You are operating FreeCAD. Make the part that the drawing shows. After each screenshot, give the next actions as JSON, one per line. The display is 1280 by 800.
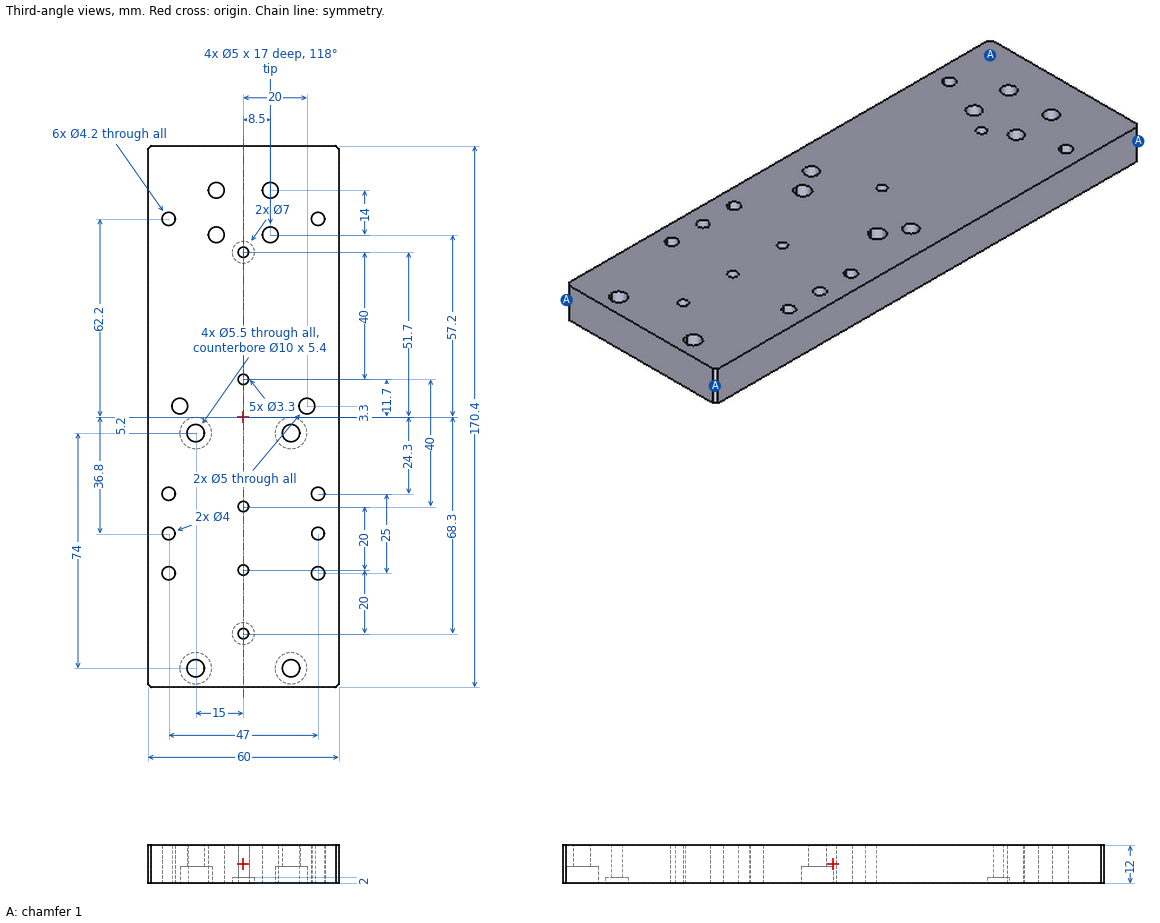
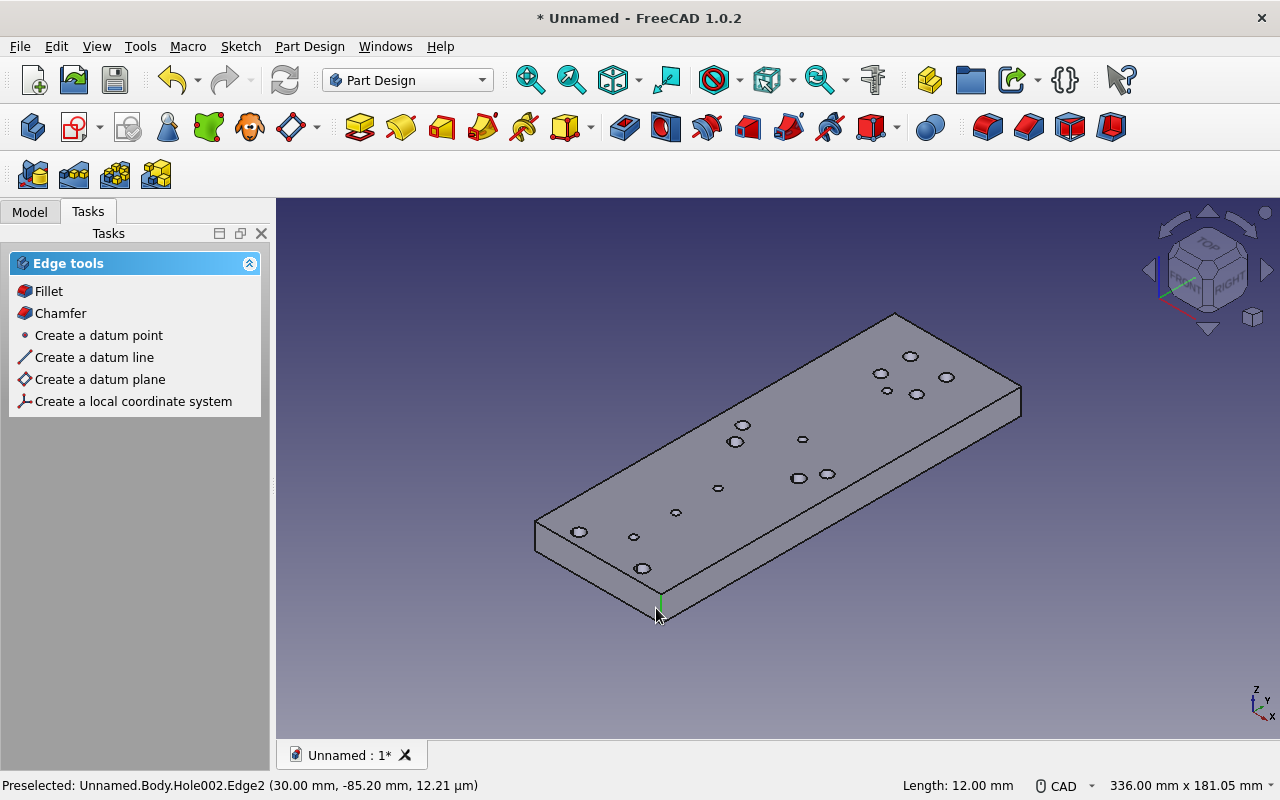
{"action": "key", "text": "1"}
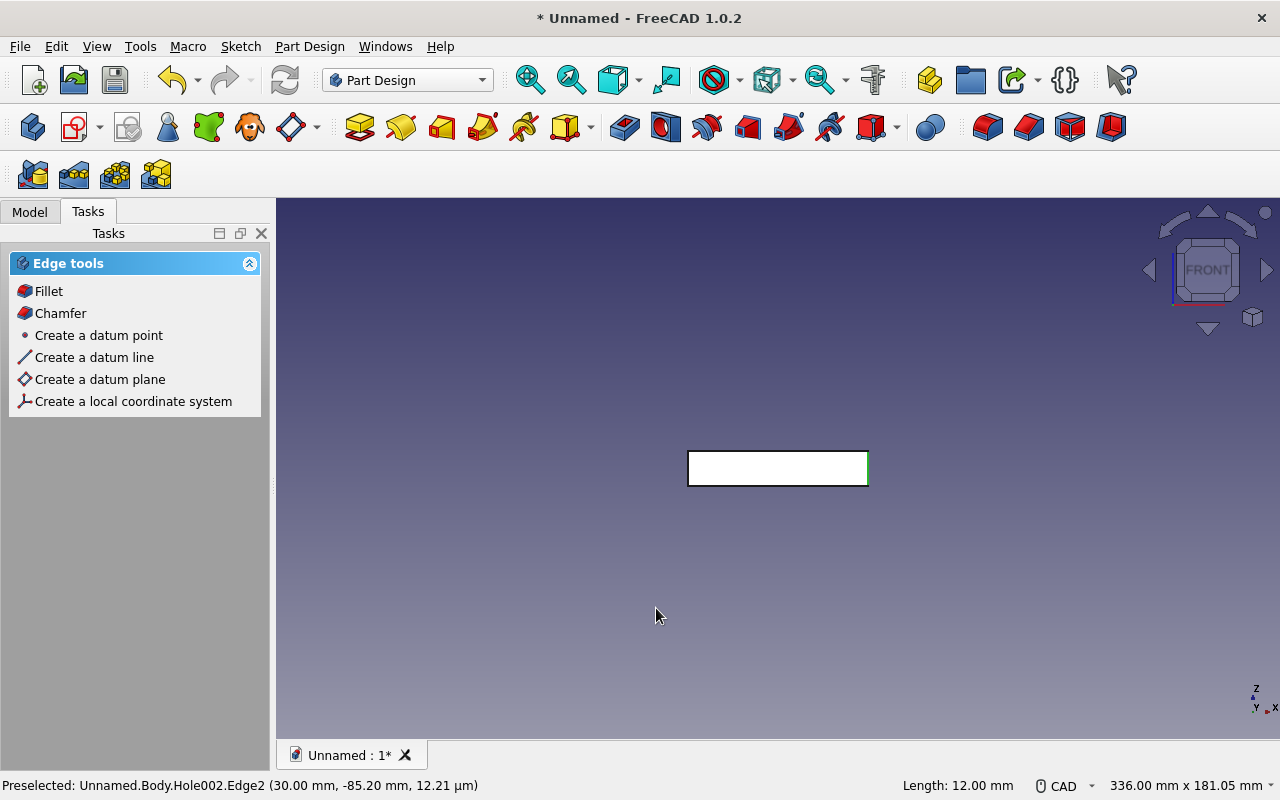
{"action": "left_click", "coordinate": [531, 80]}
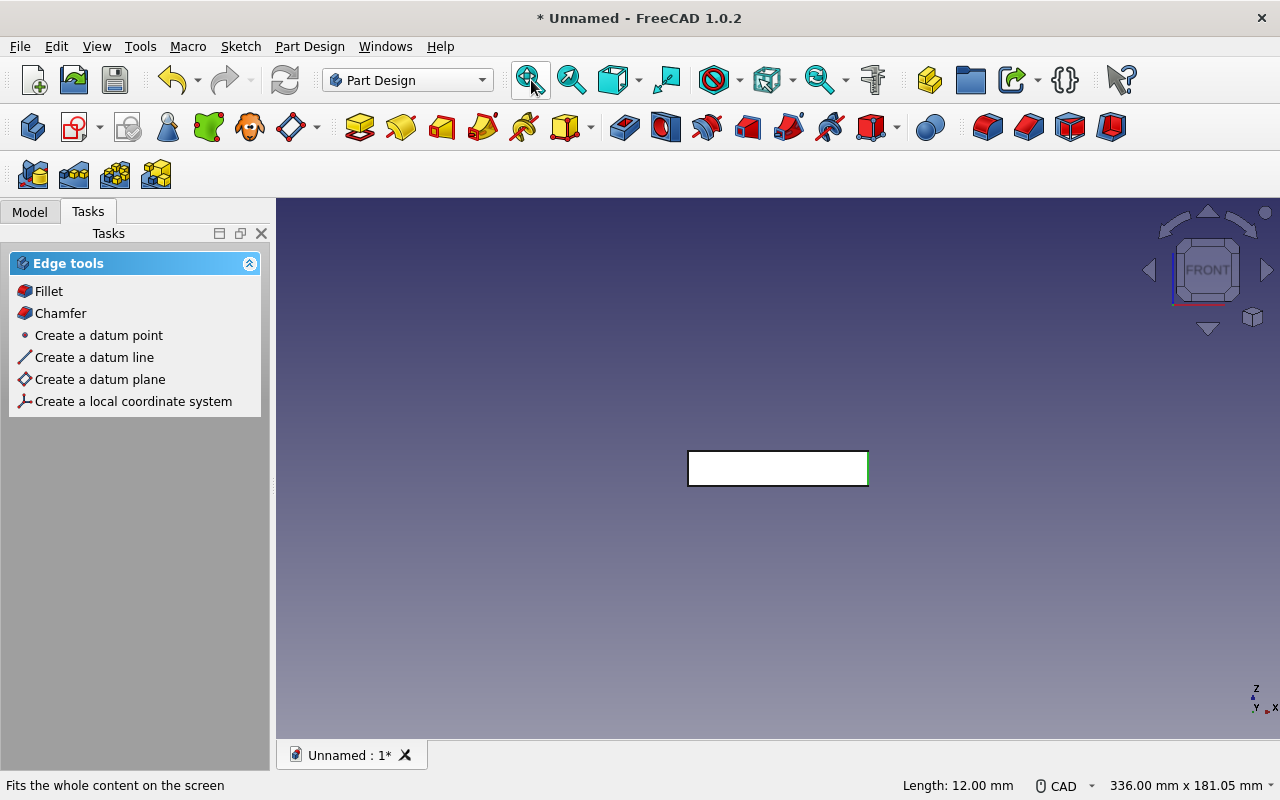
{"action": "left_click", "coordinate": [688, 468], "text": "ctrl"}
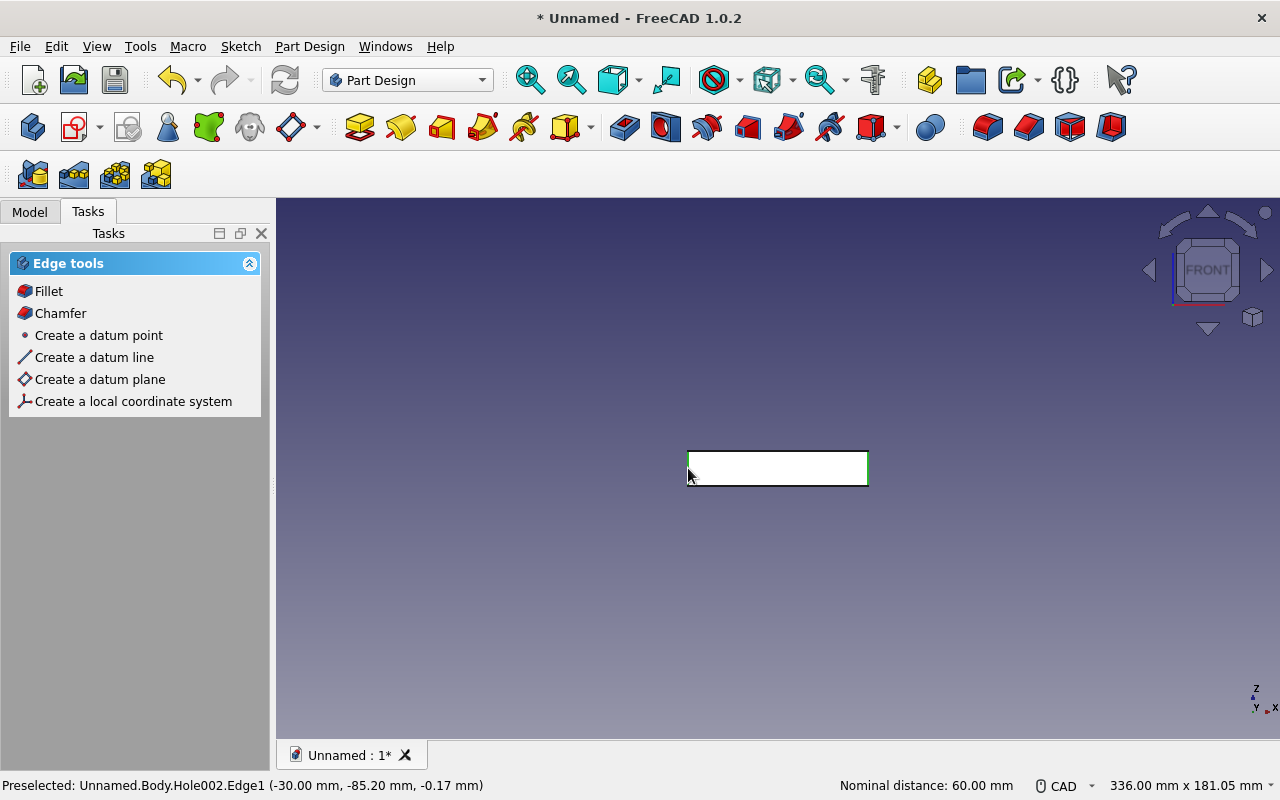
{"action": "key", "text": "3"}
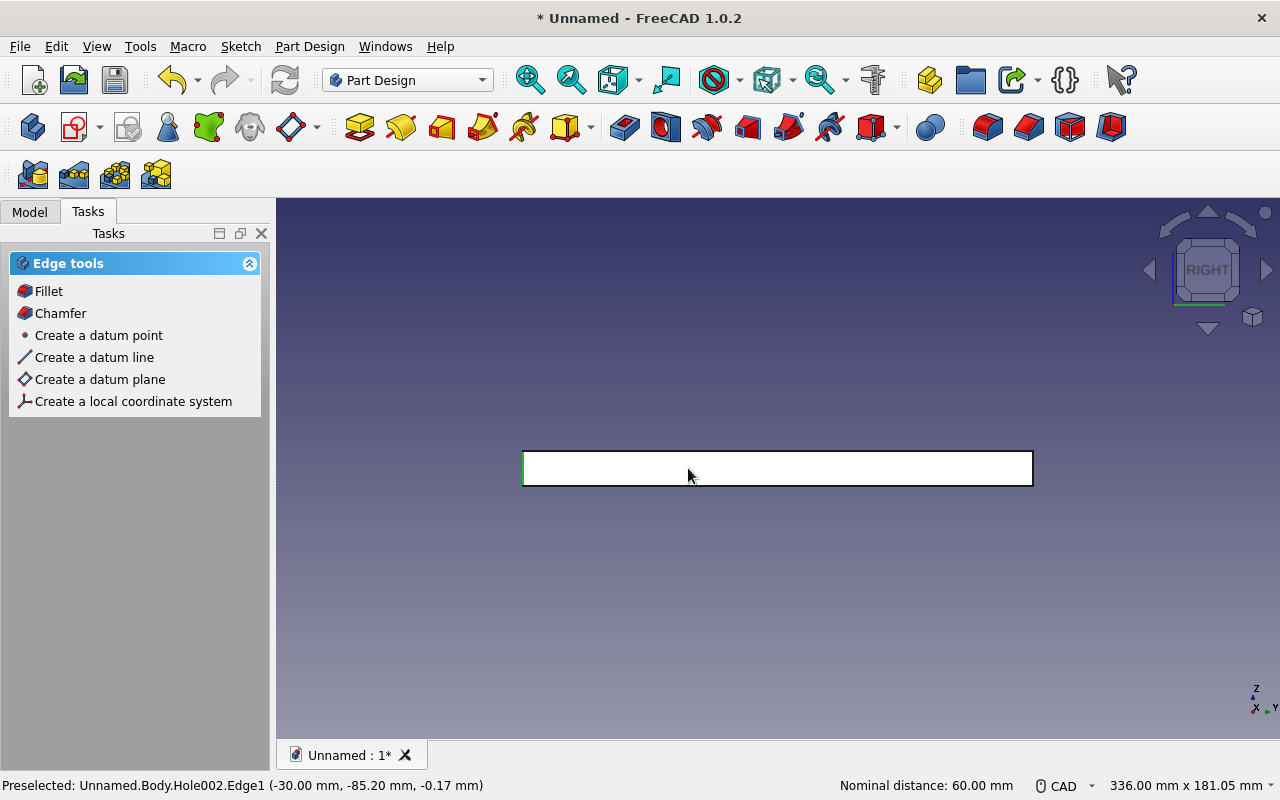
{"action": "left_click", "coordinate": [1033, 467], "text": "ctrl"}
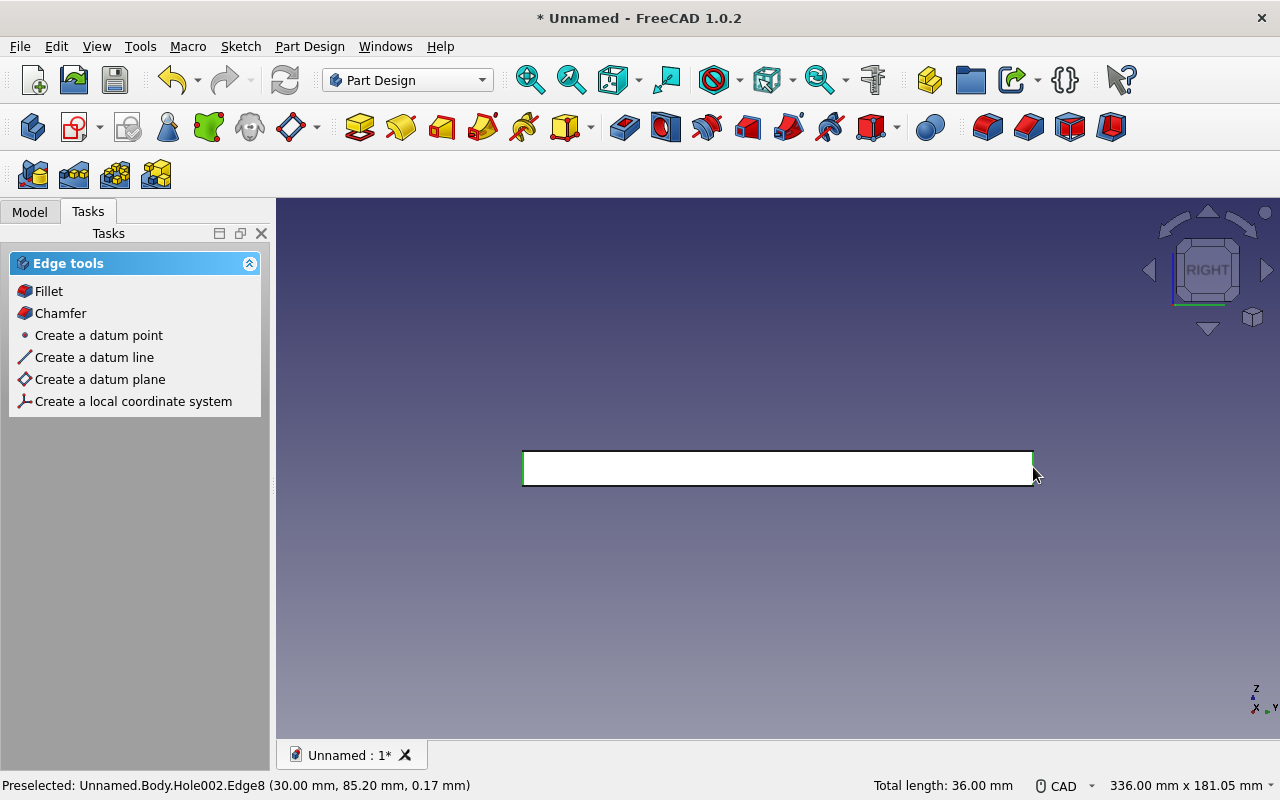
{"action": "key", "text": "5"}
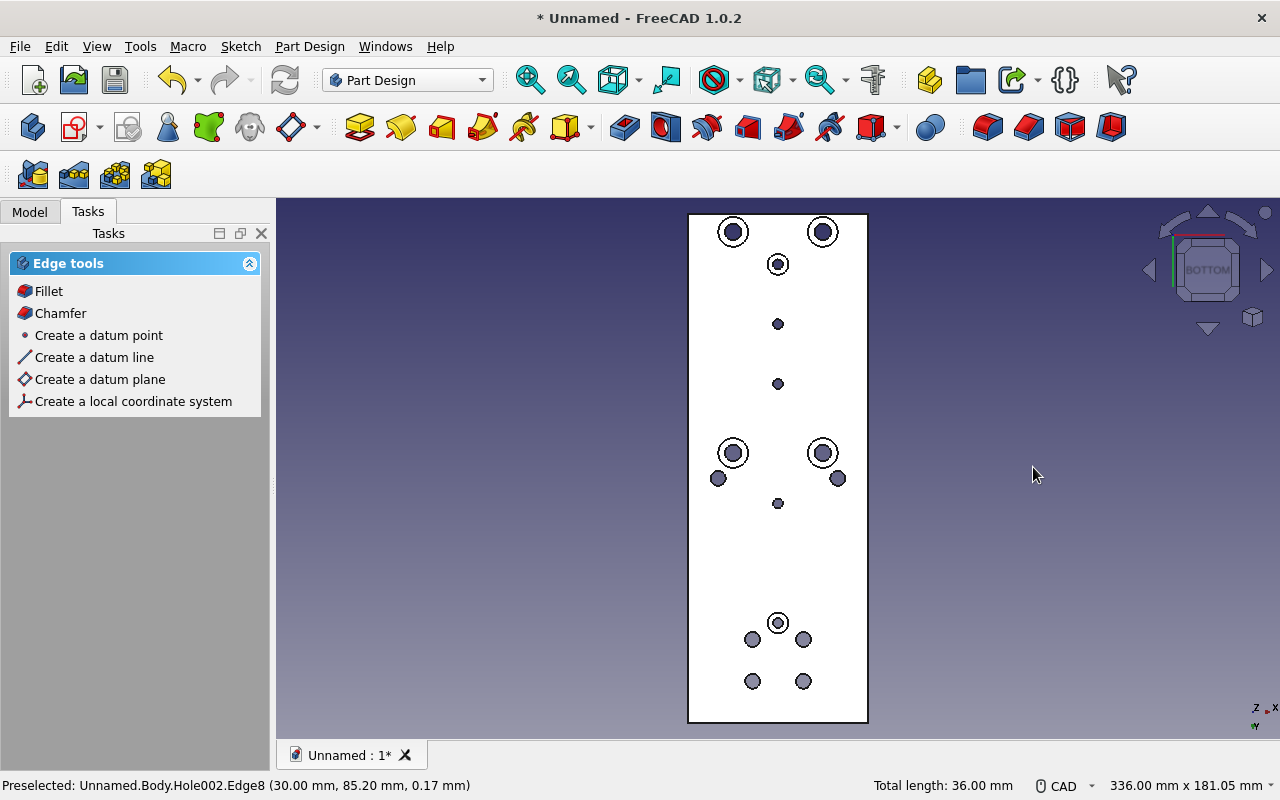
{"action": "key", "text": "4"}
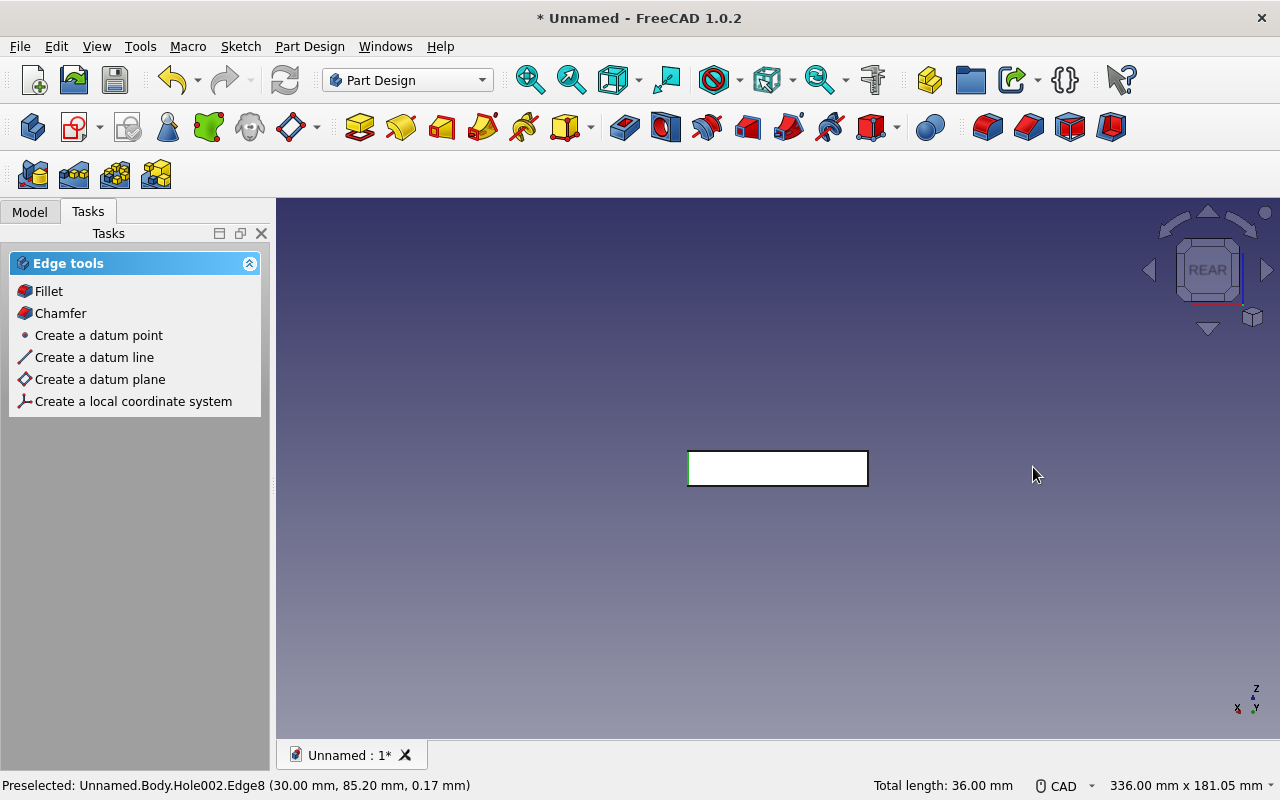
{"action": "left_click", "coordinate": [531, 80]}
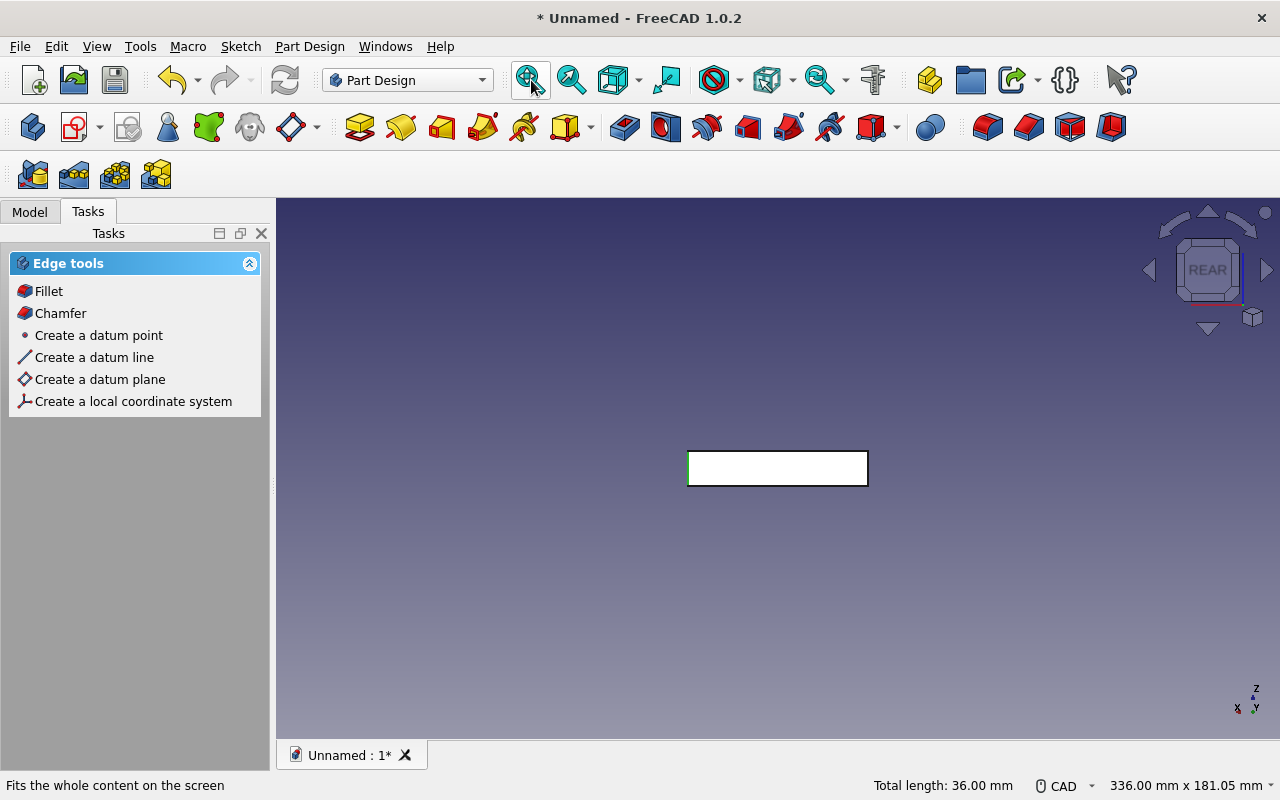
{"action": "left_click", "coordinate": [868, 468], "text": "ctrl"}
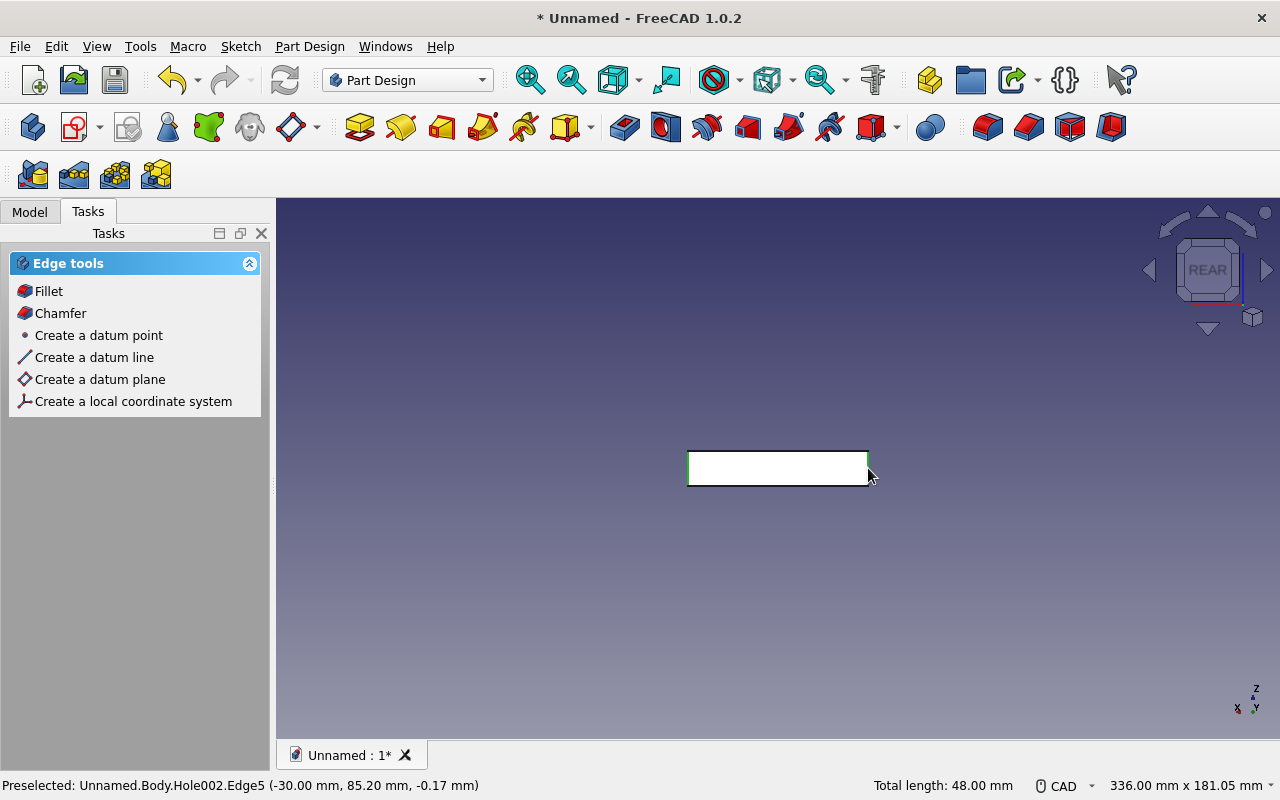
{"action": "left_click", "coordinate": [1029, 128]}